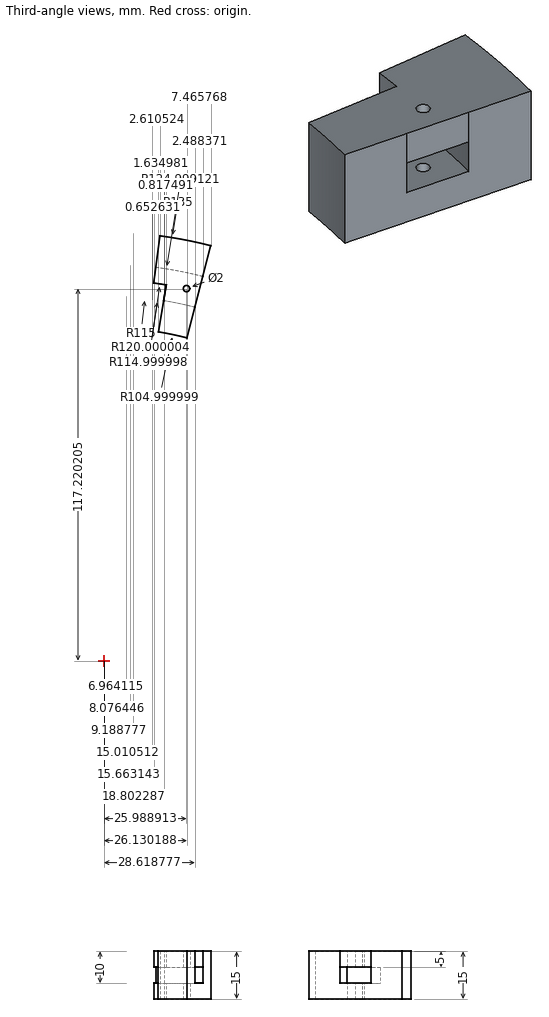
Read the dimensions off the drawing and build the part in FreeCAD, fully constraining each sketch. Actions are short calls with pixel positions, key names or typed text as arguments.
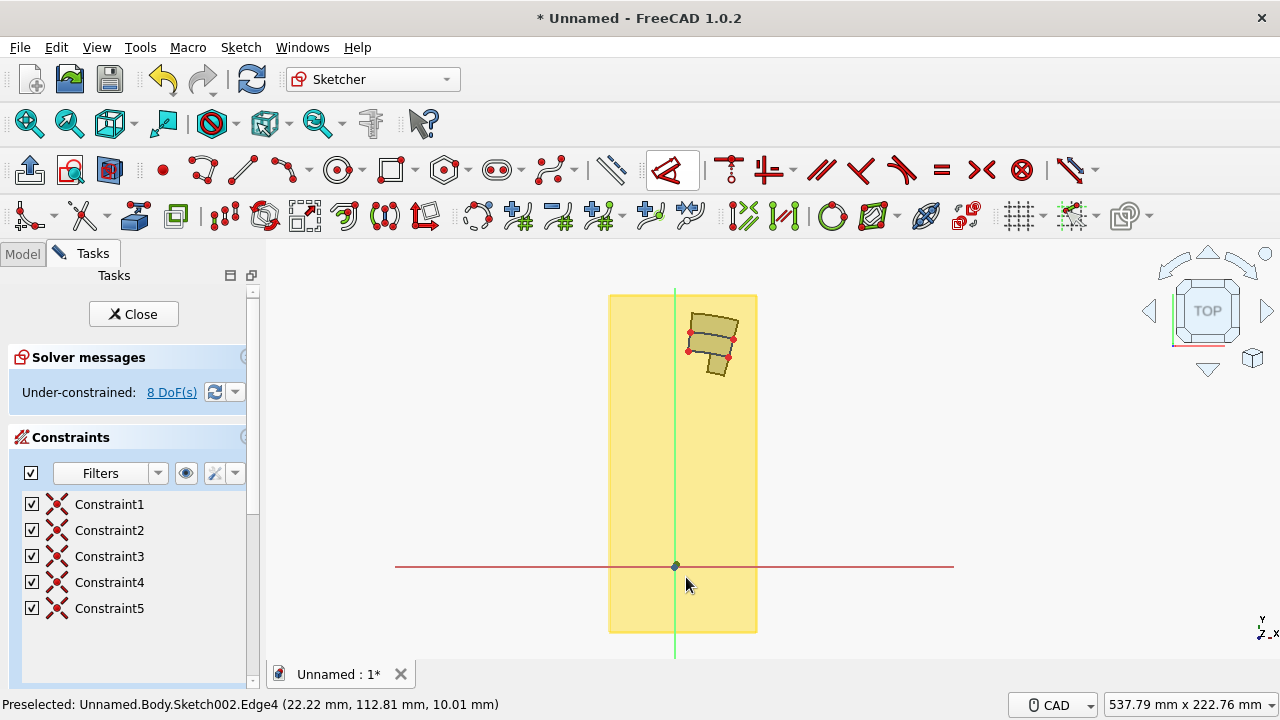
click(730, 170)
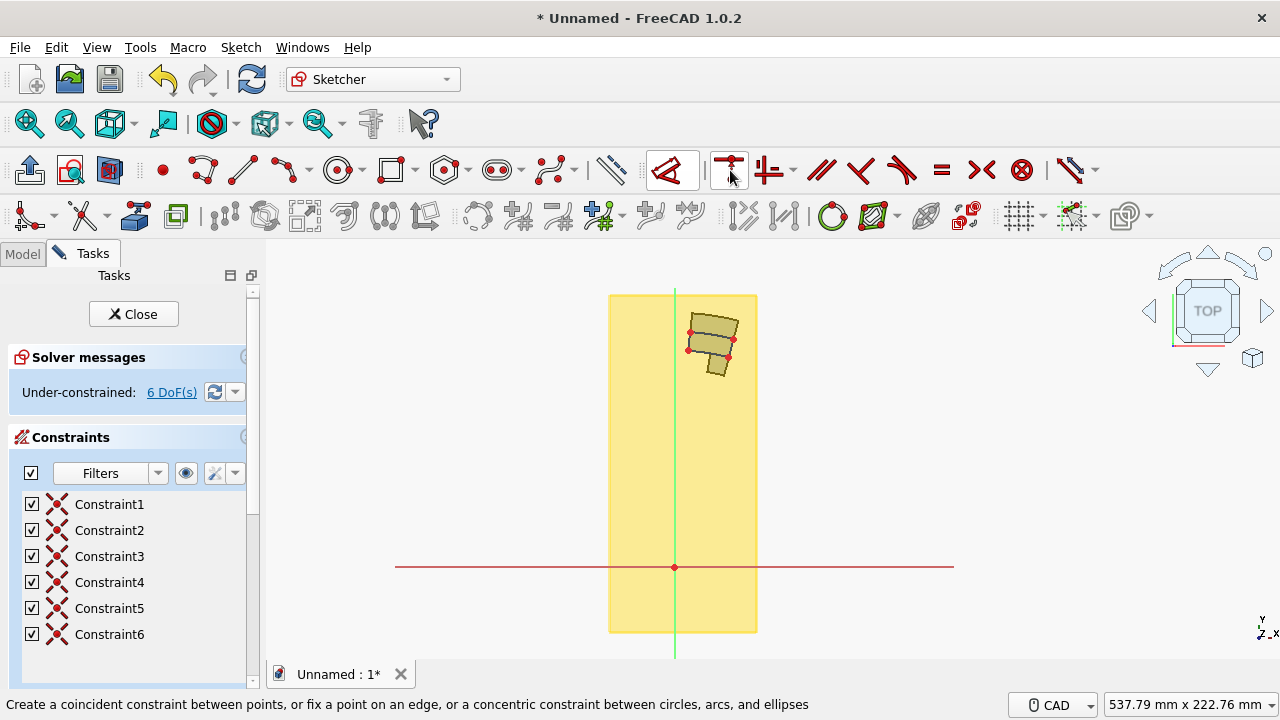
click(721, 336)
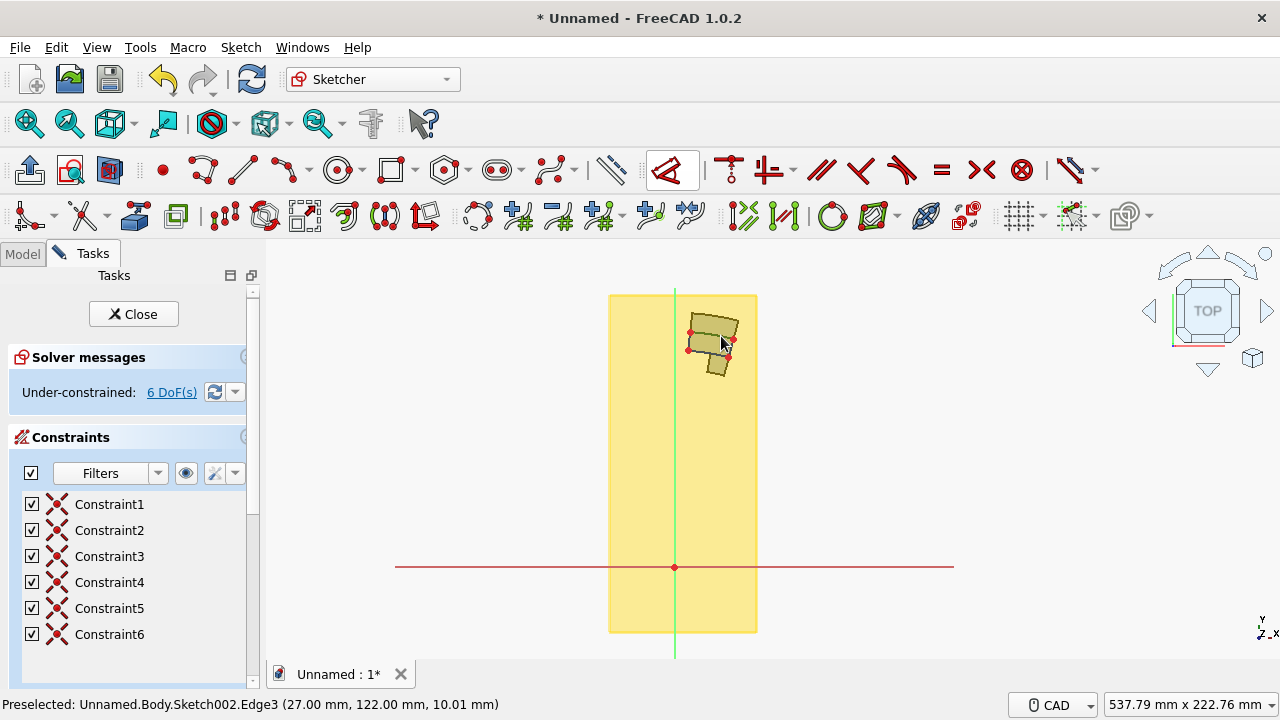
key(k)
key(r)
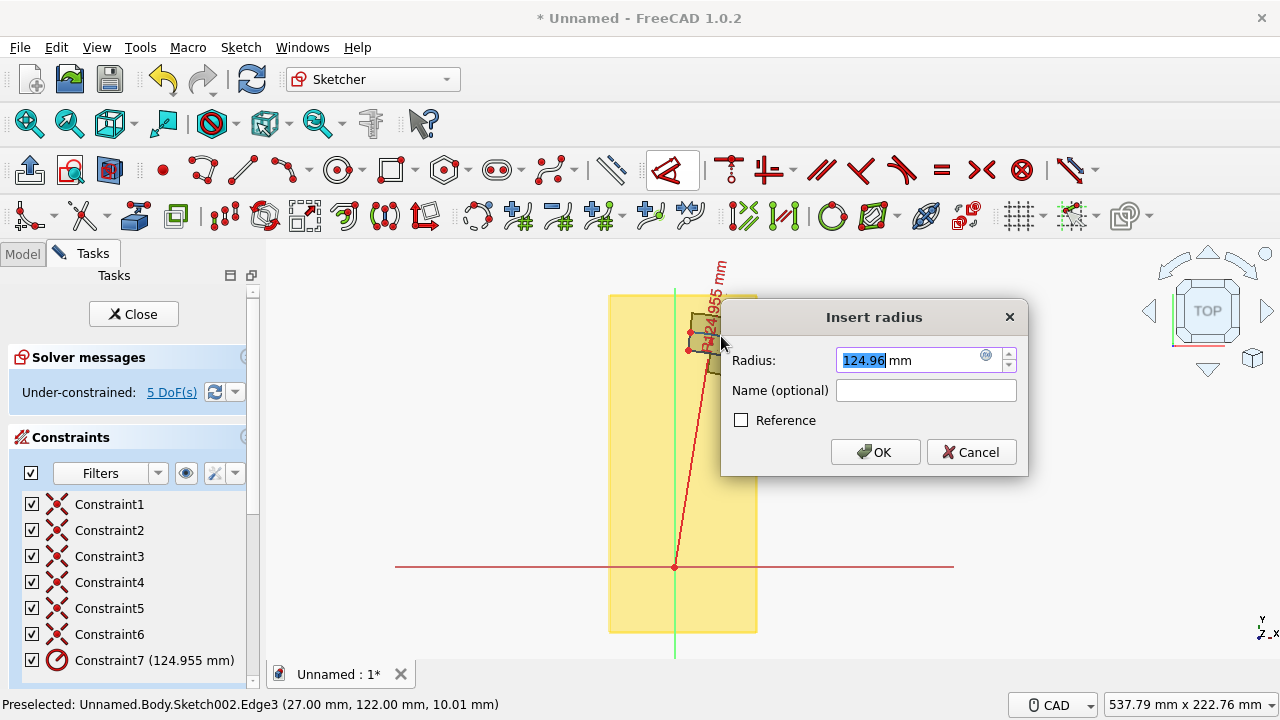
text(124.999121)
key(Return)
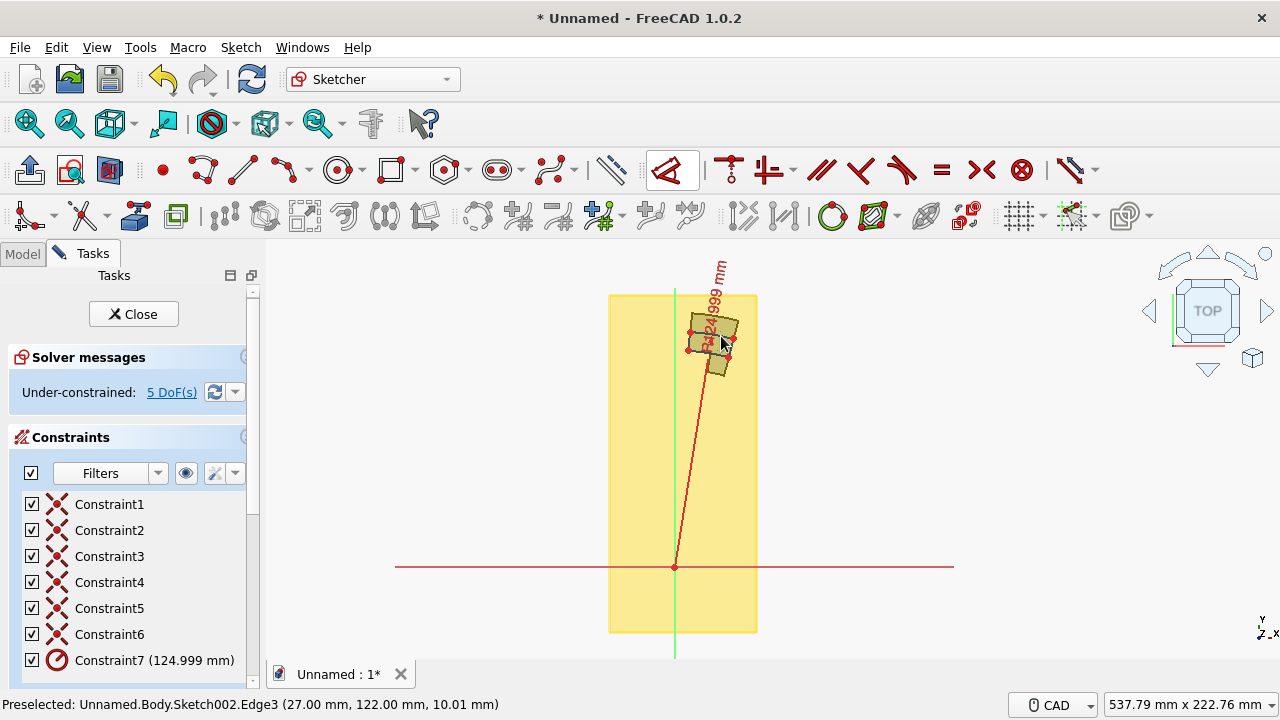
click(717, 355)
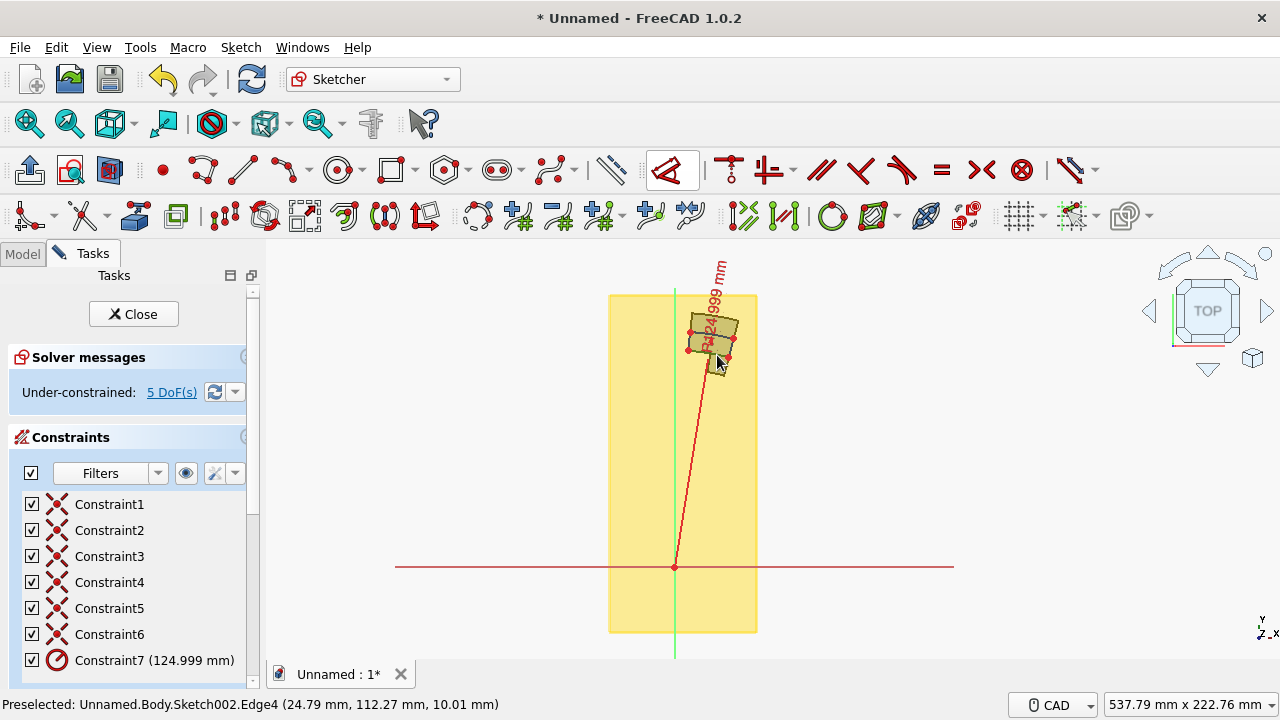
click(694, 170)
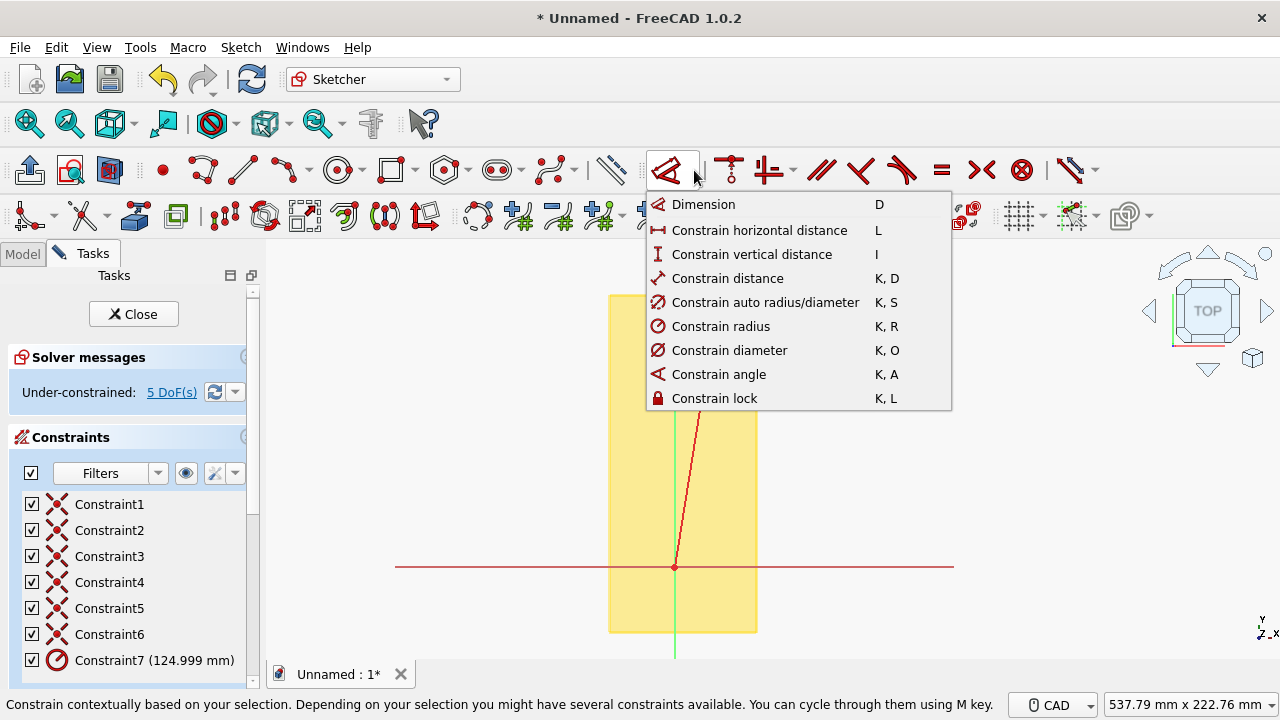
click(799, 326)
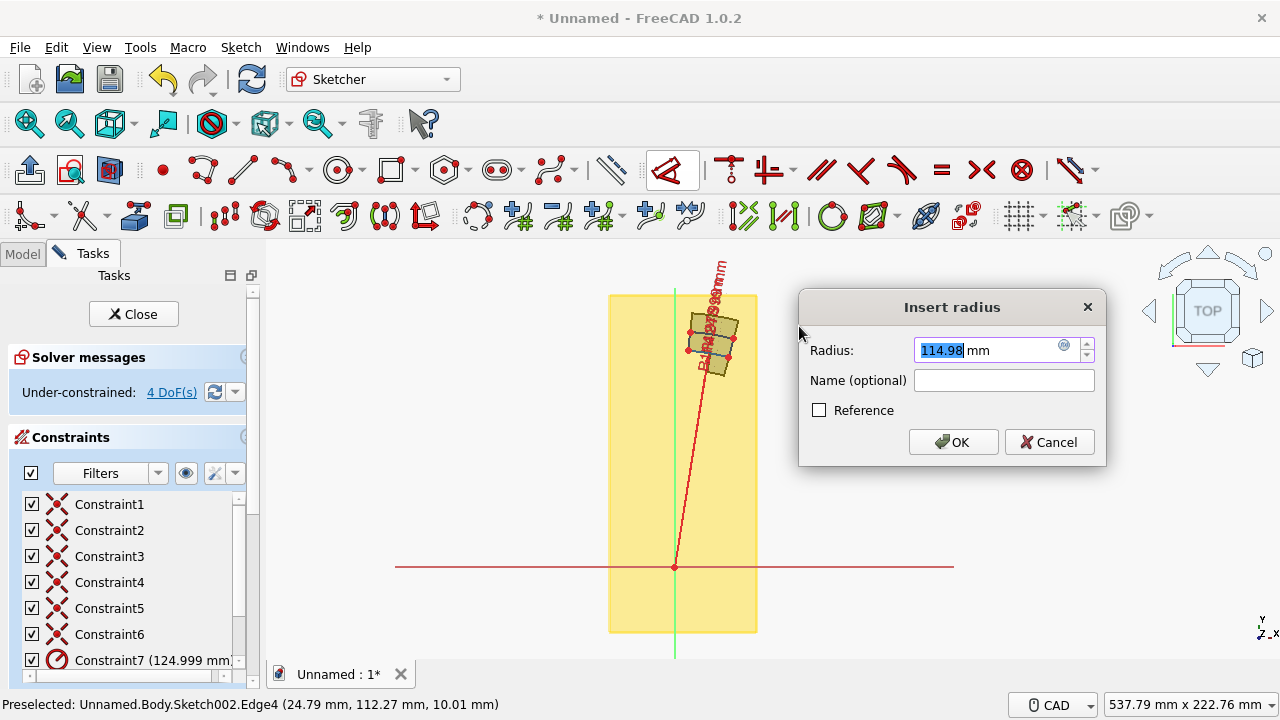
text(115)
key(Return)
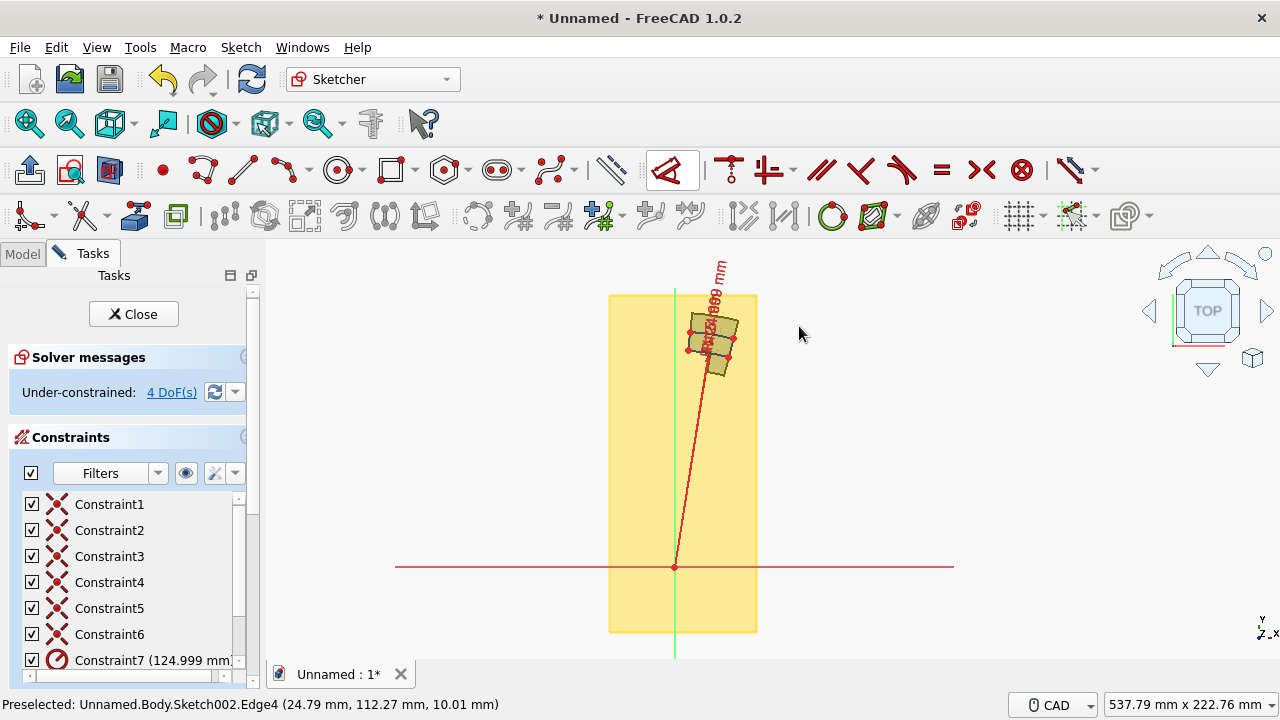
scroll(690, 332, up, 5)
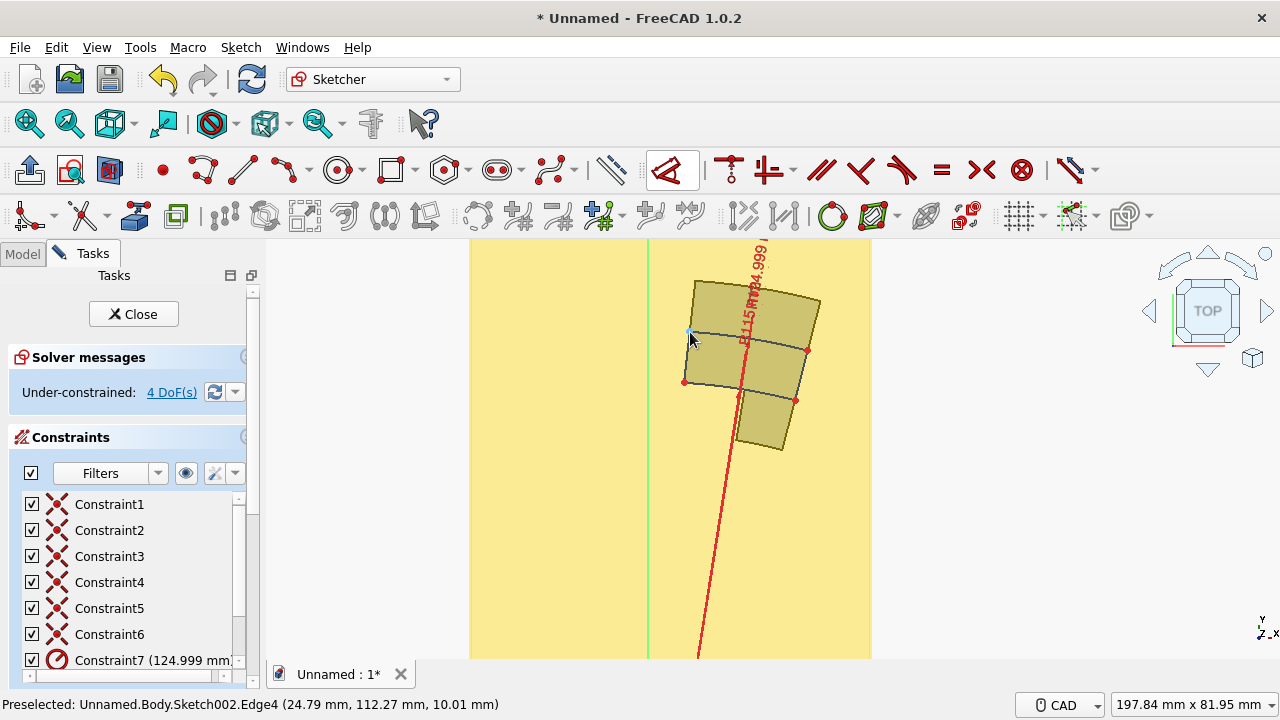
click(690, 332)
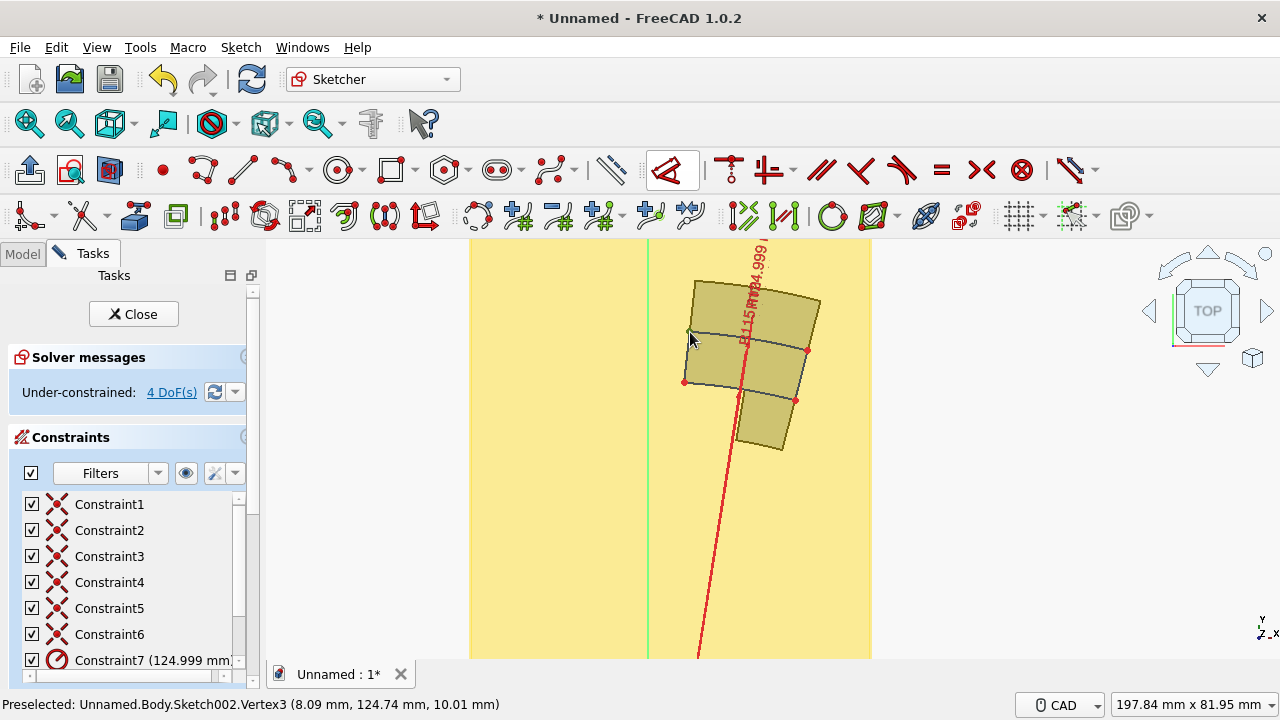
click(694, 170)